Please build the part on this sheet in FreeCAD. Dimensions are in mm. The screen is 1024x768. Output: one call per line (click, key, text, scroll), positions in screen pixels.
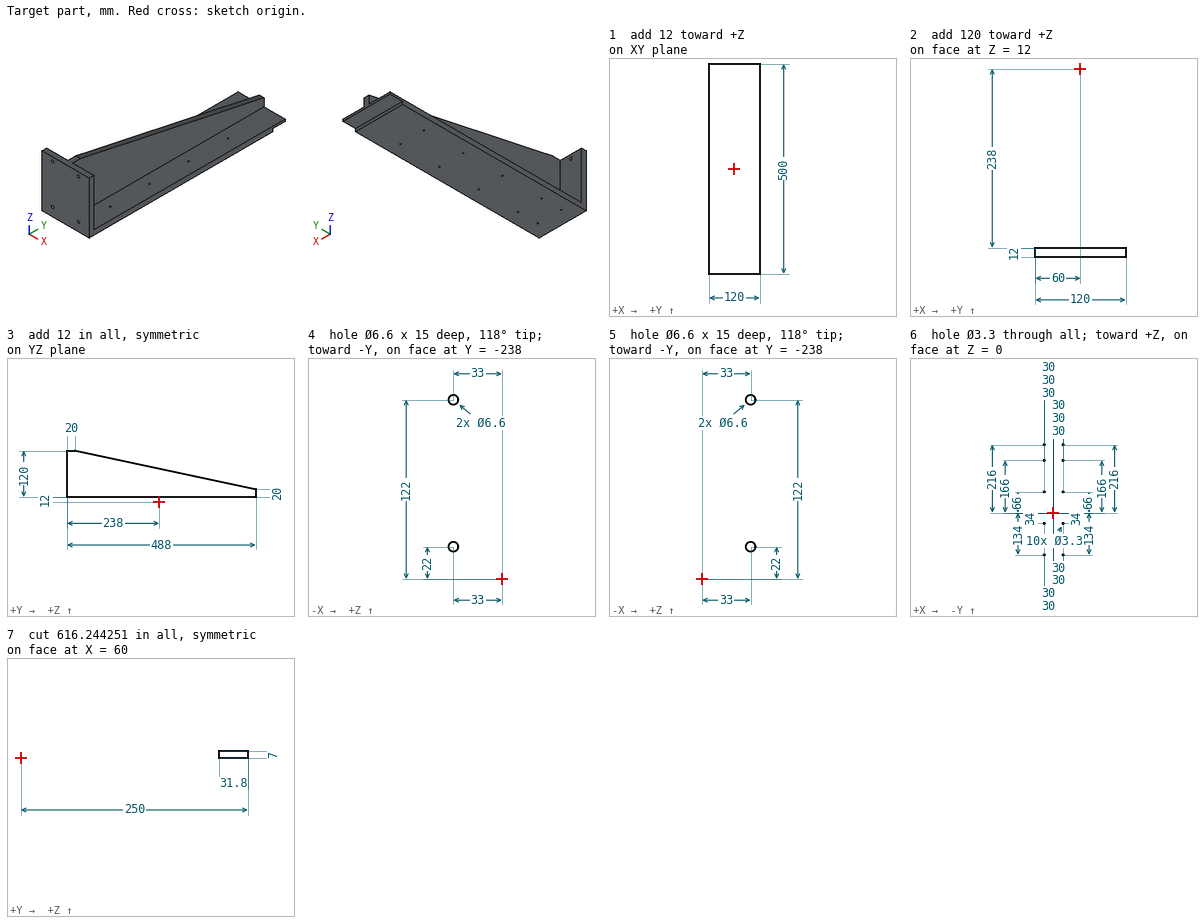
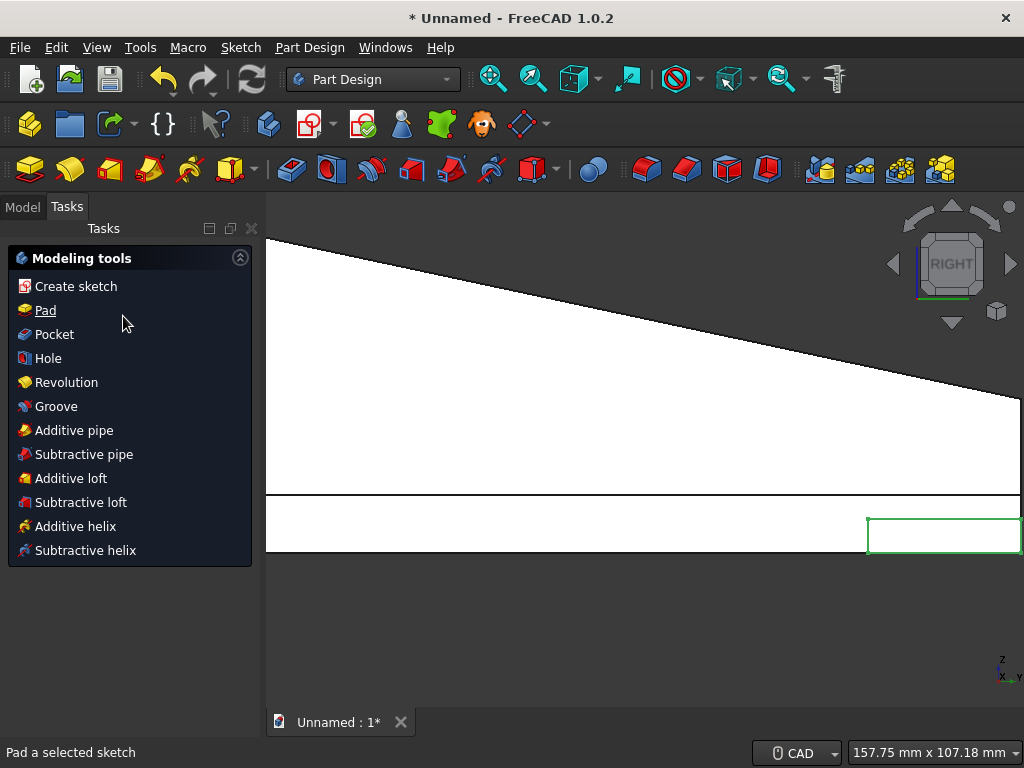
click(292, 170)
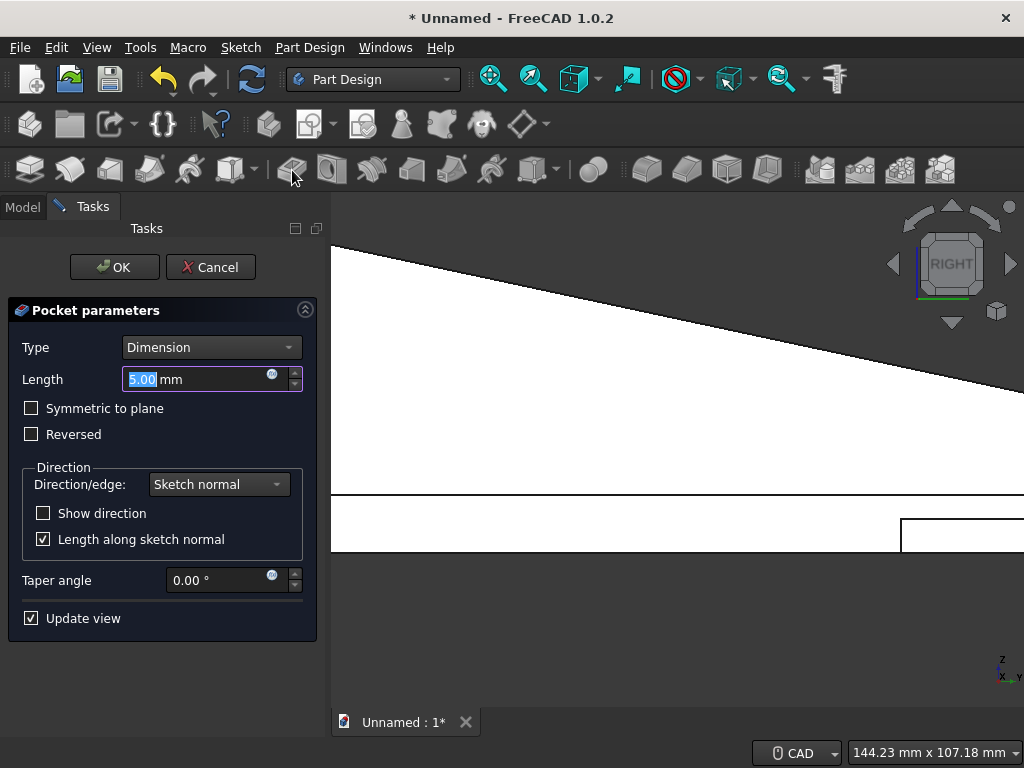
text(616.244251)
key(Tab)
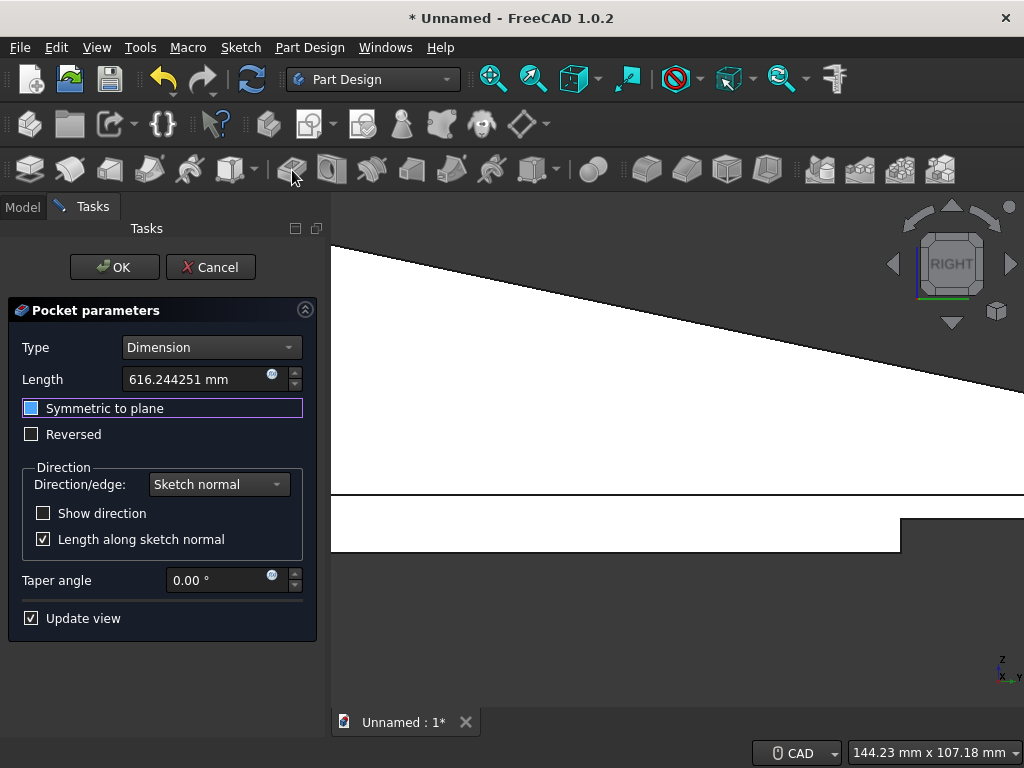
click(30, 408)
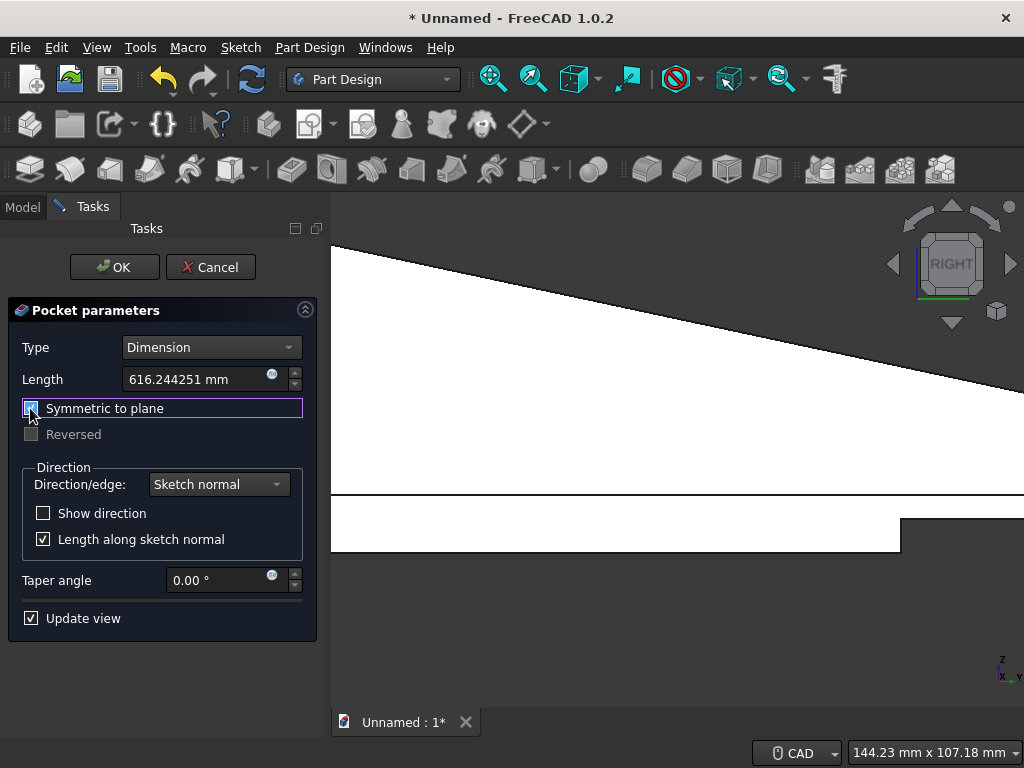
click(115, 267)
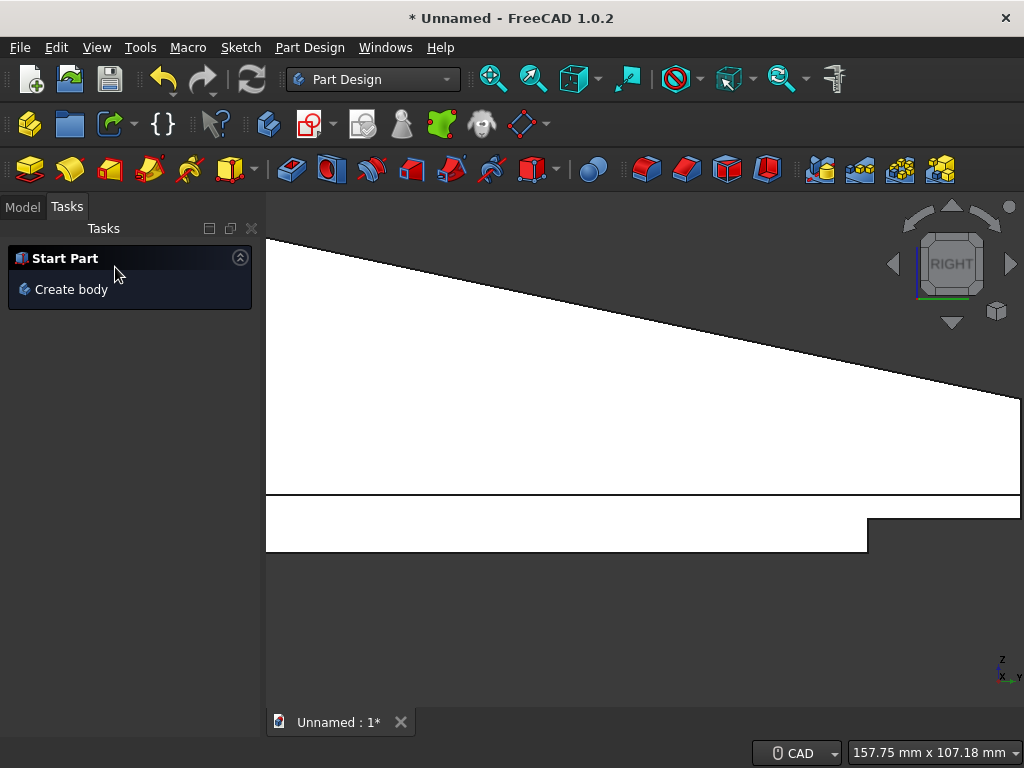
key(0)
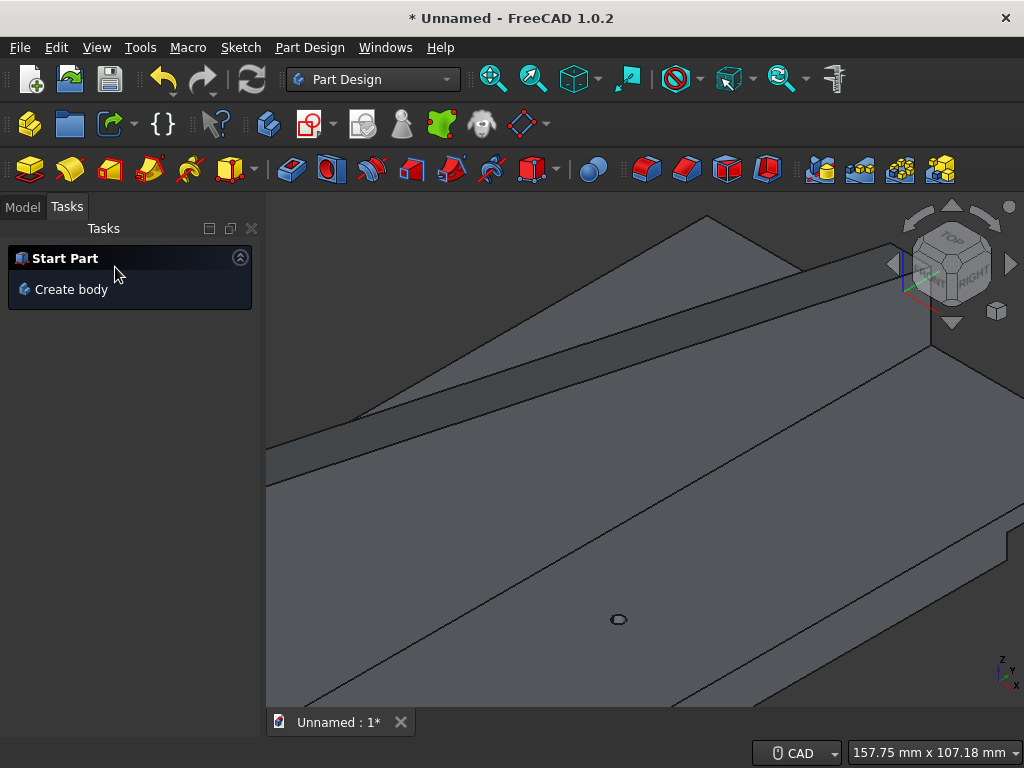
click(494, 80)